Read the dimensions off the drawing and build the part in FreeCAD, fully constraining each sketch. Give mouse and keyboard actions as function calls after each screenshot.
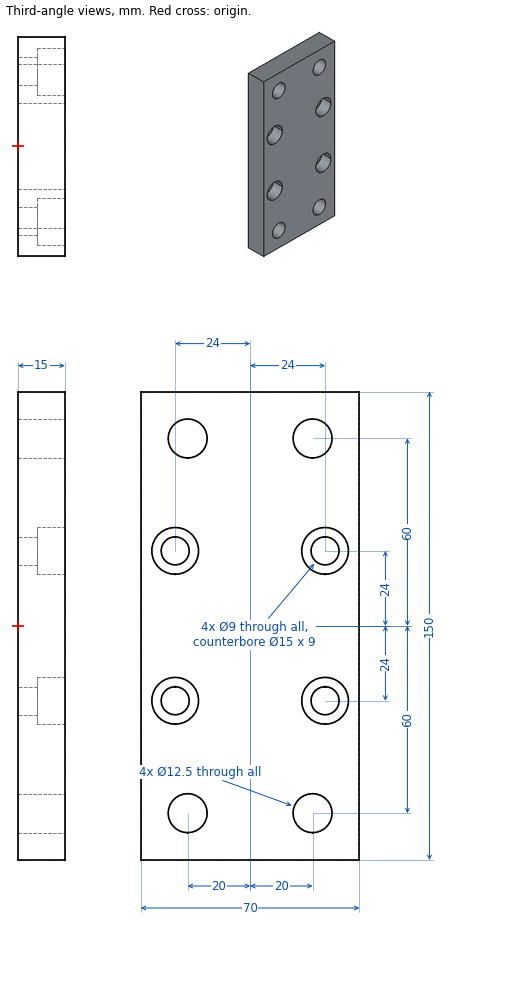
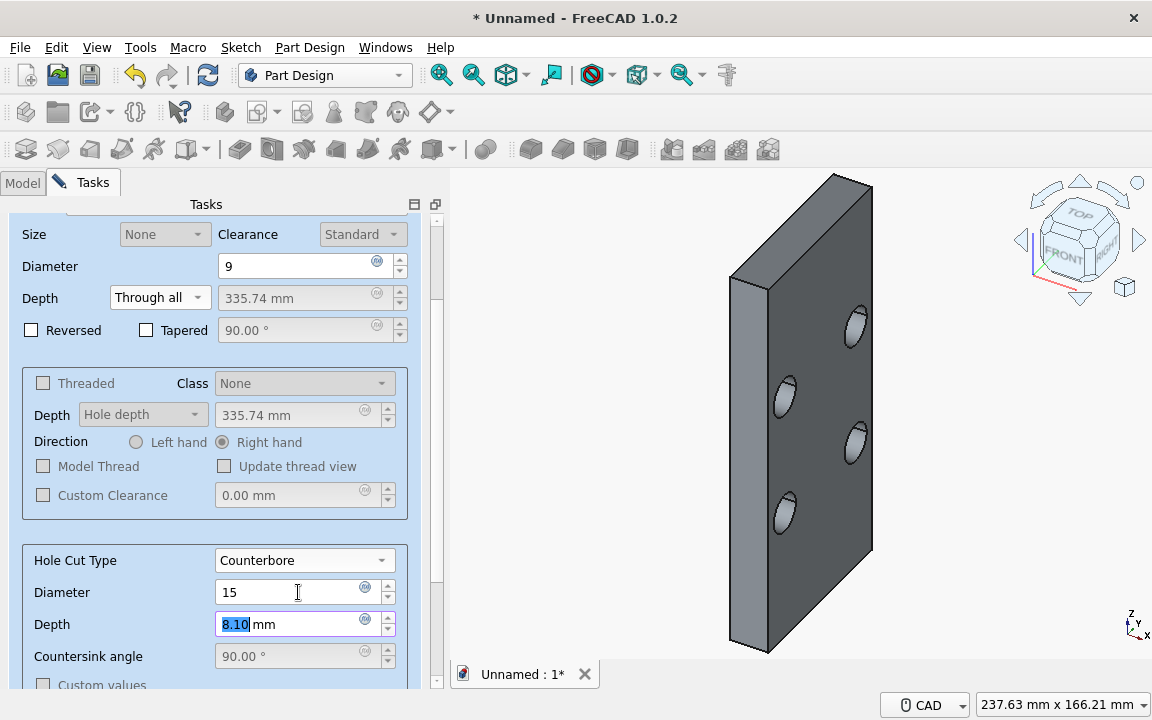
text(9)
key(Tab)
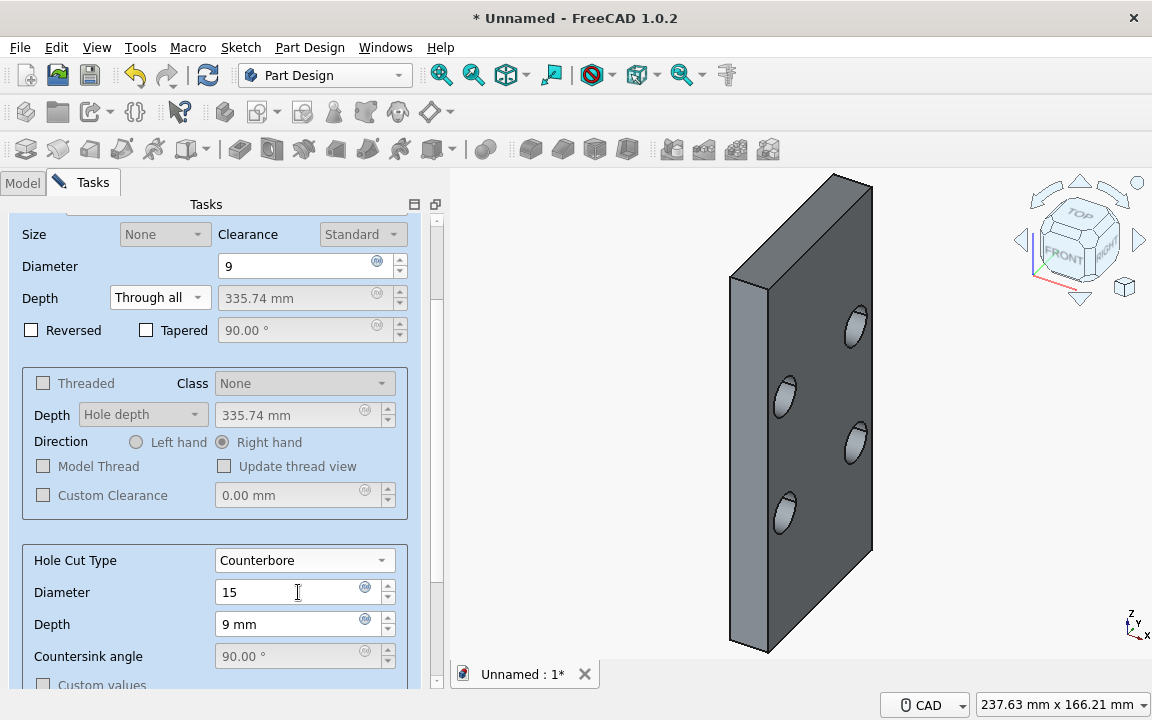
scroll(437, 451, up, 3)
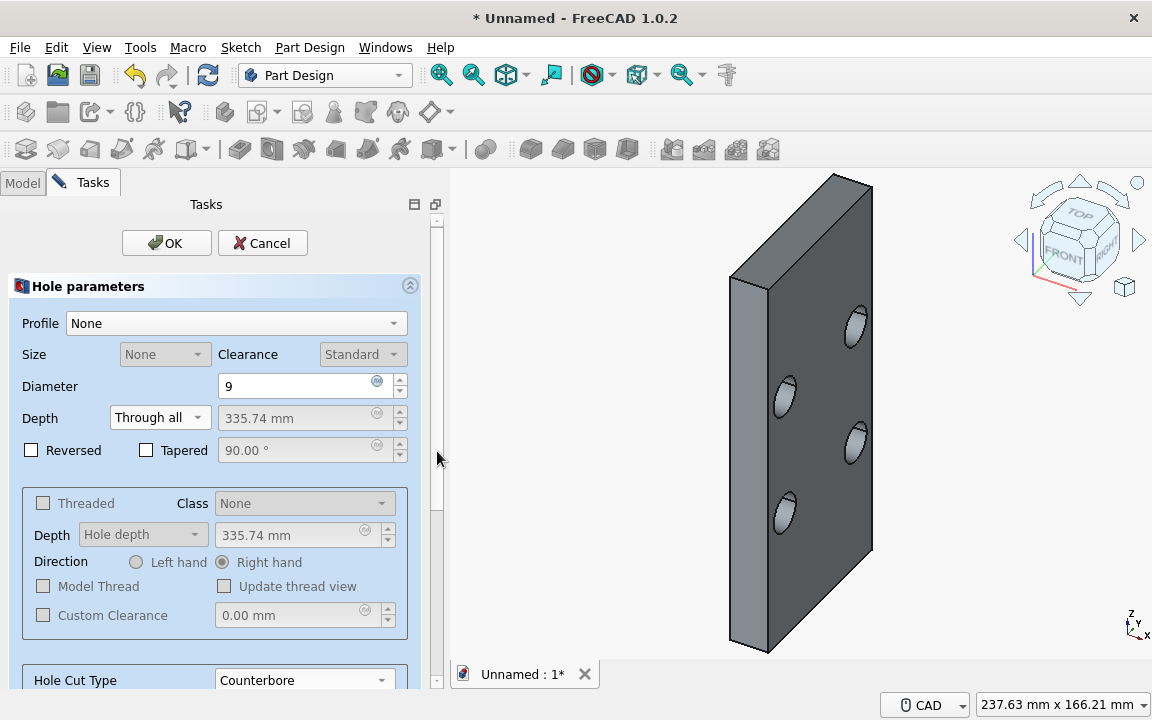
click(167, 243)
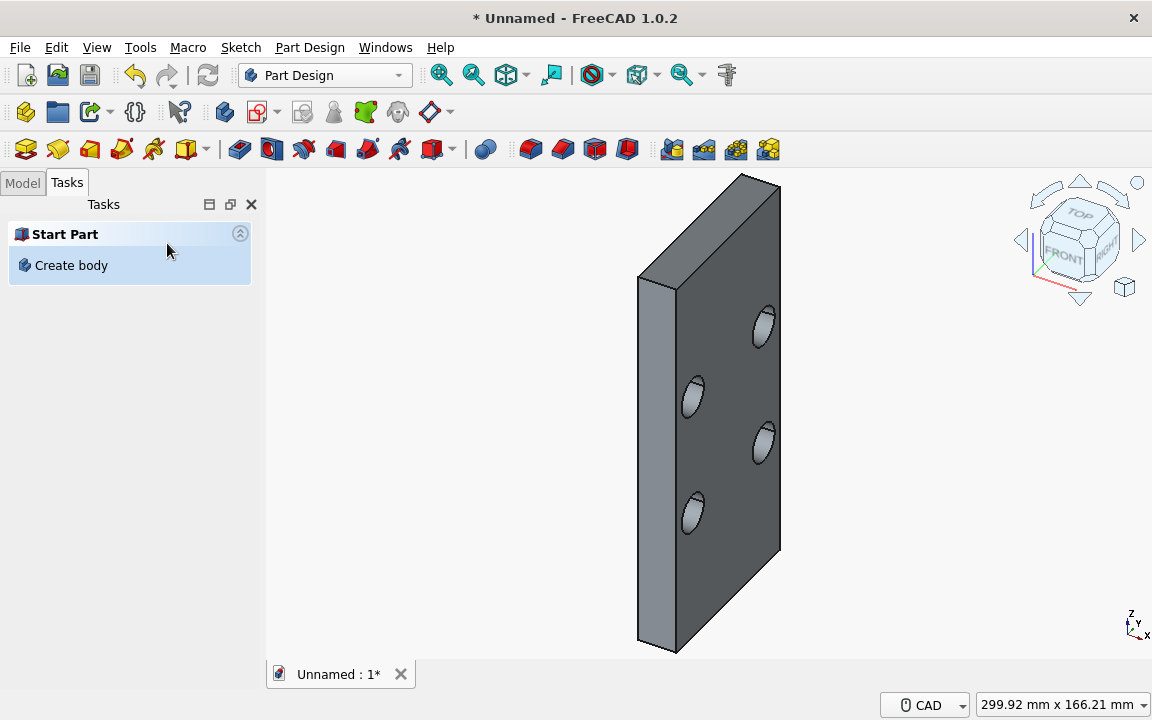
click(258, 112)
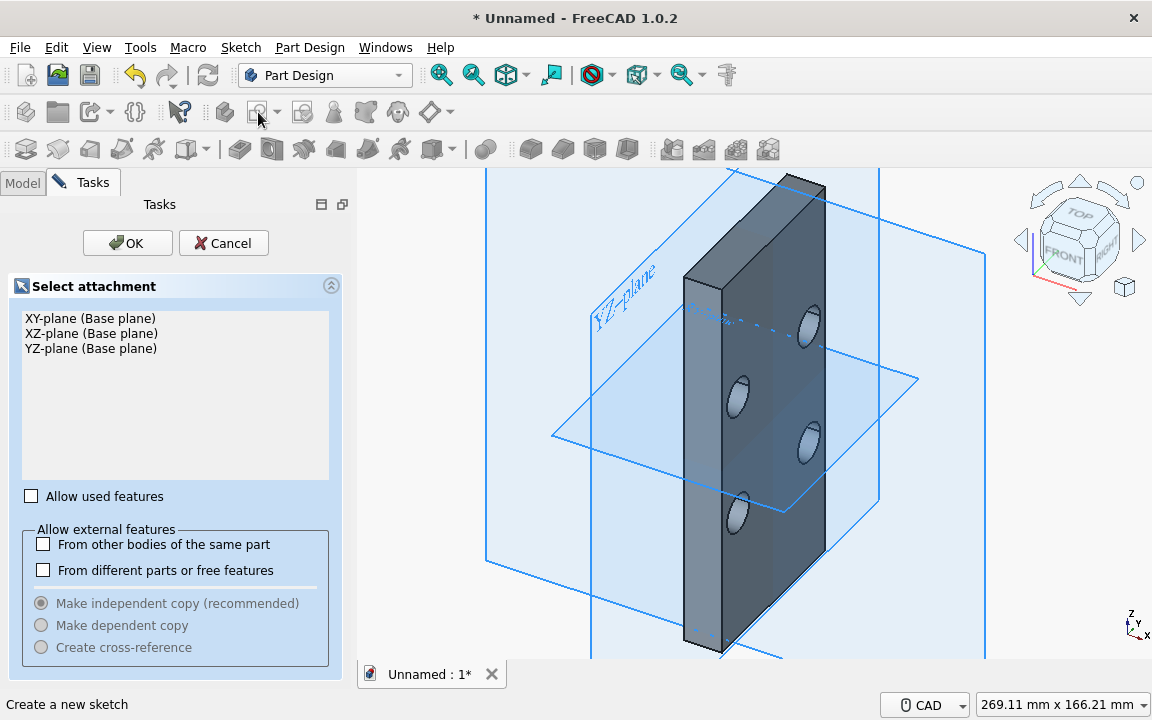
click(82, 348)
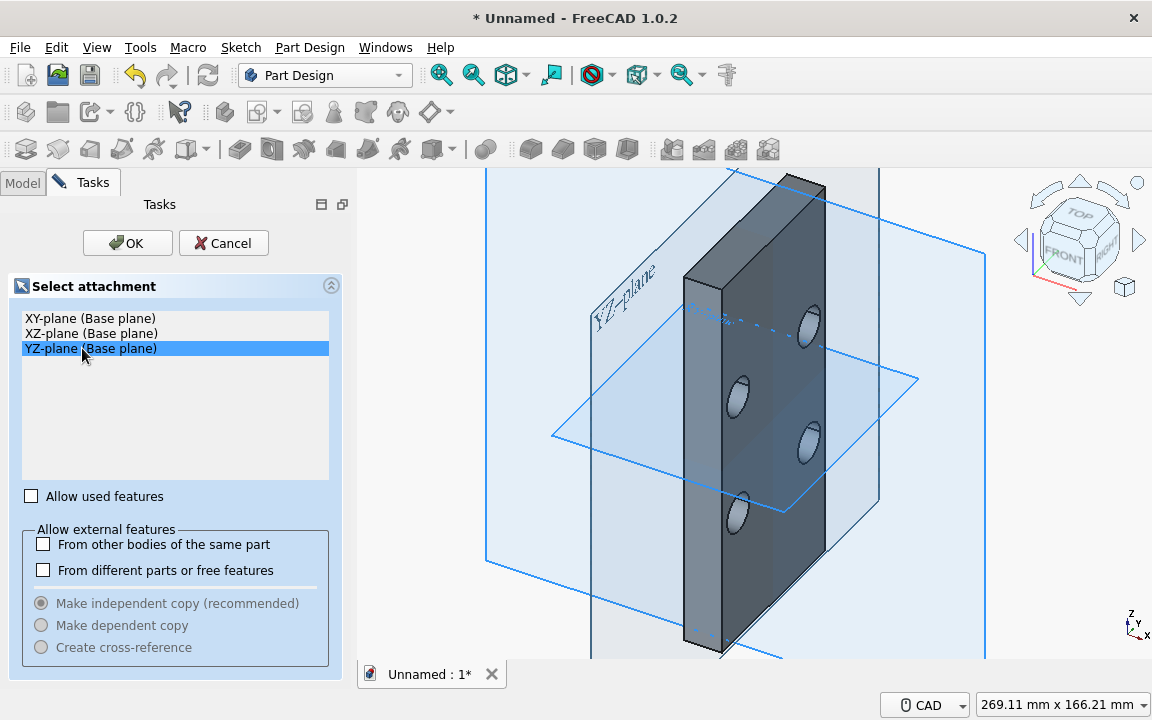
click(128, 243)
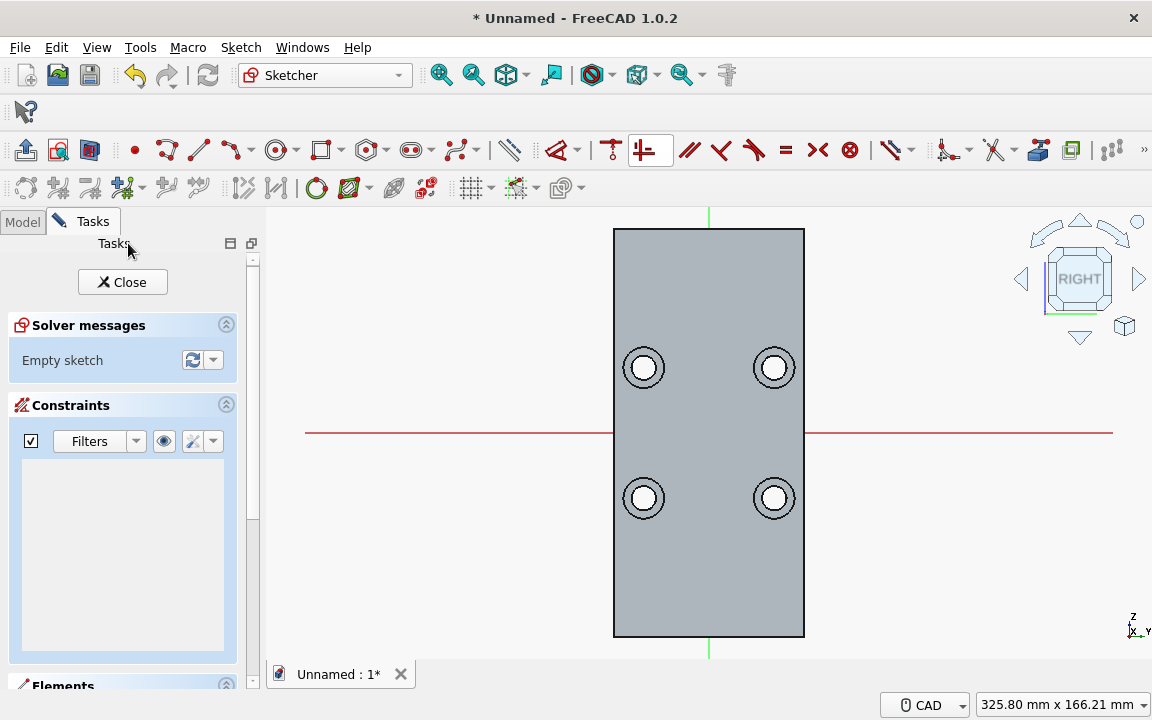
click(90, 150)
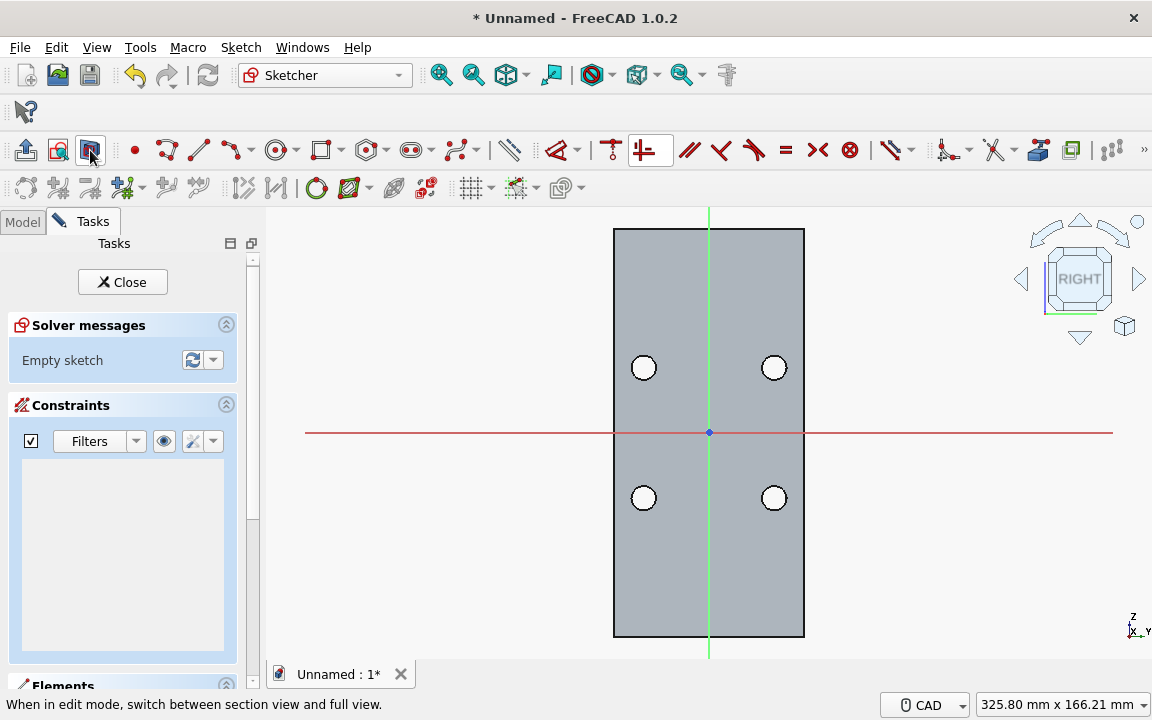
scroll(331, 433, down, 1)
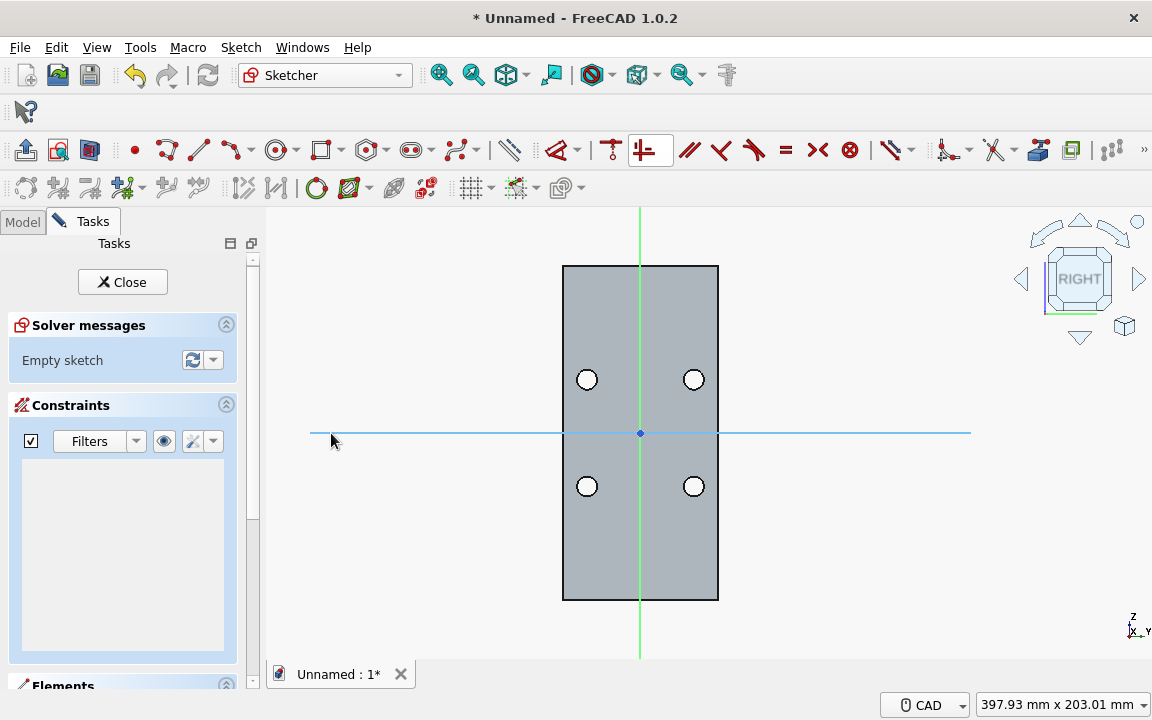
click(276, 150)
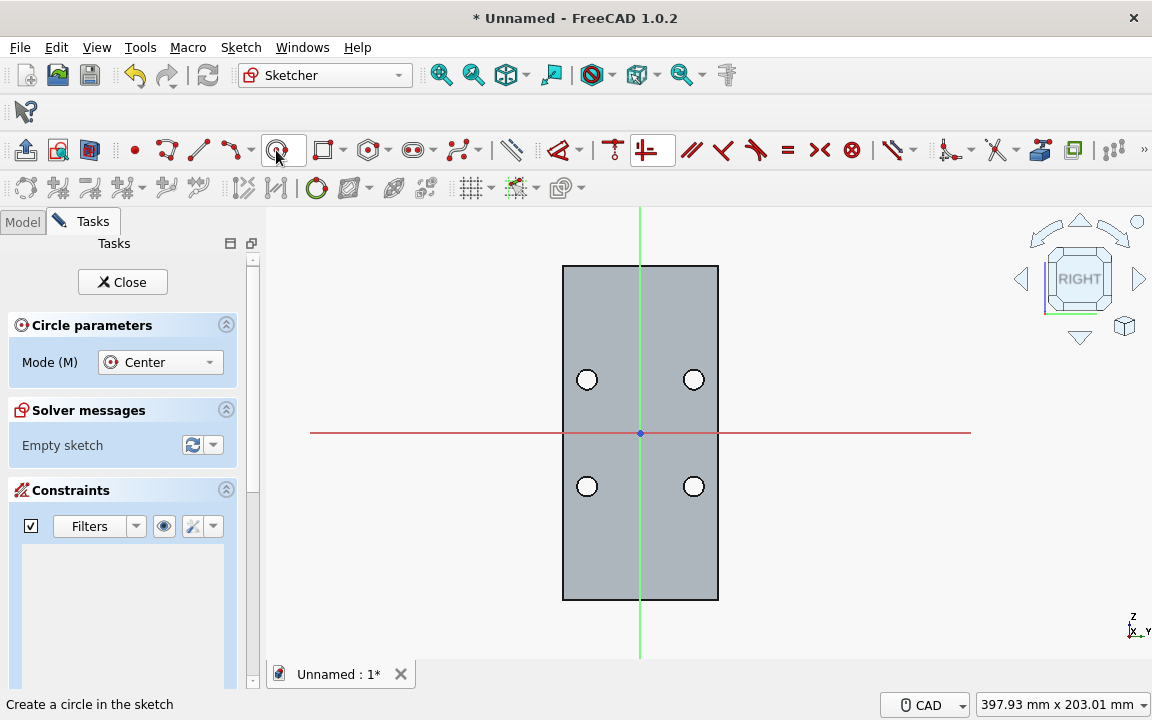
scroll(685, 567, up, 3)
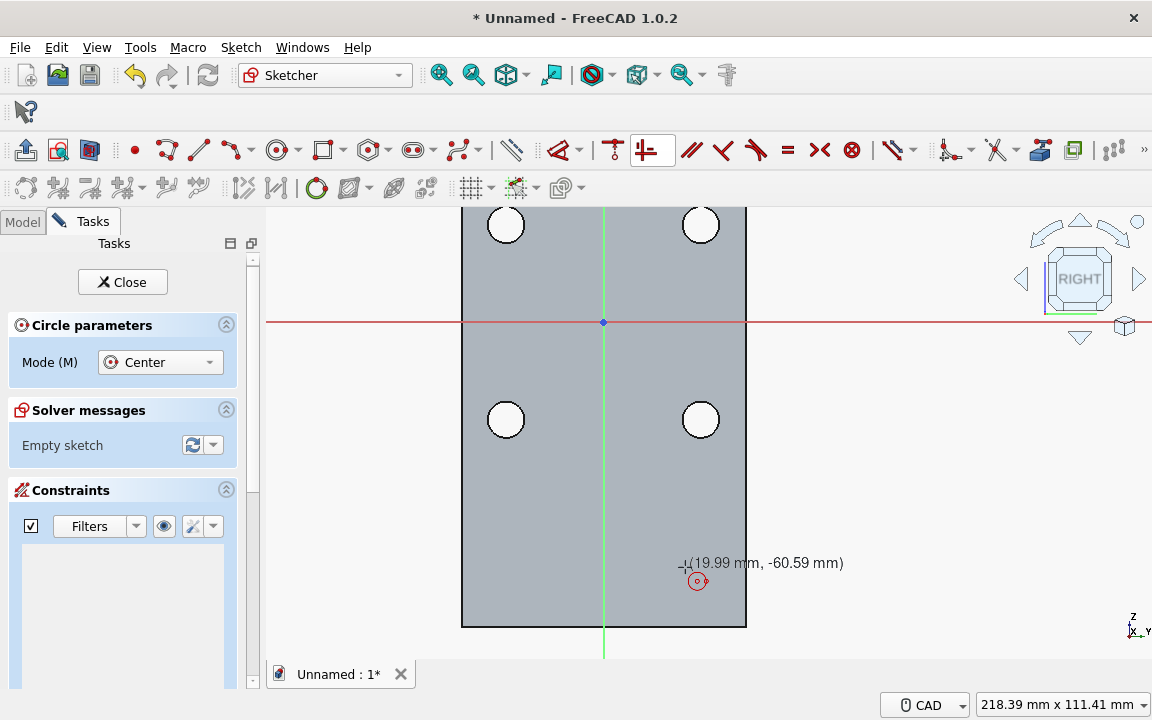
click(685, 566)
click(703, 548)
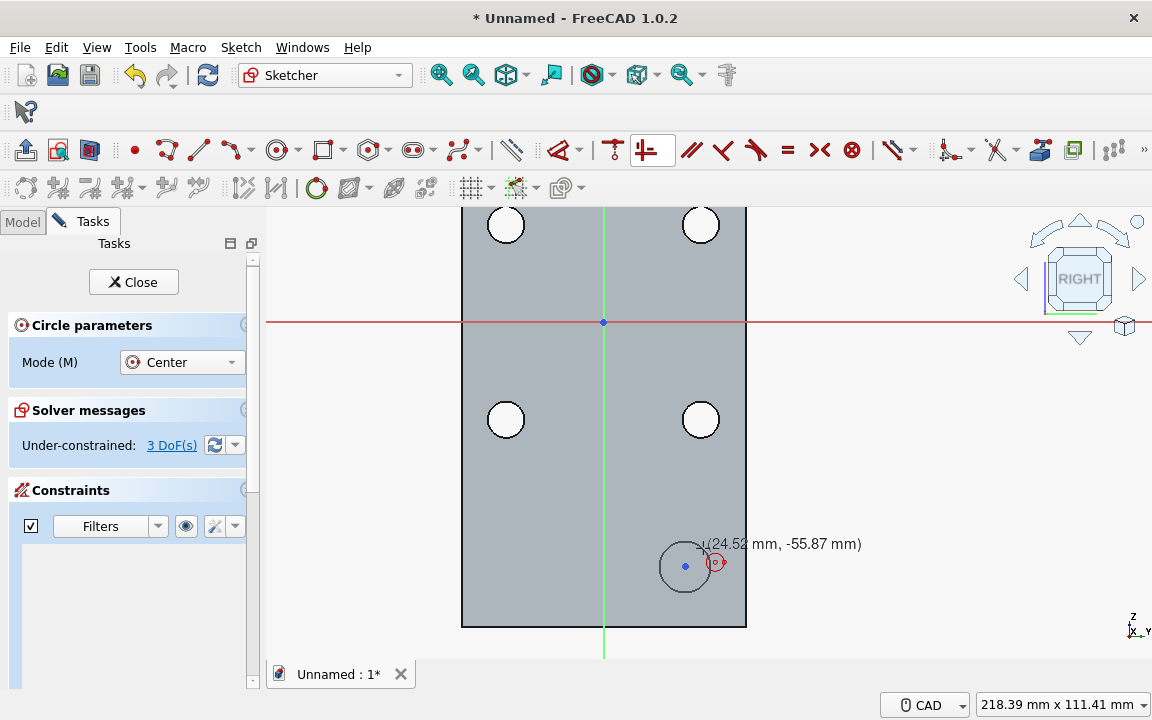
click(522, 566)
click(540, 548)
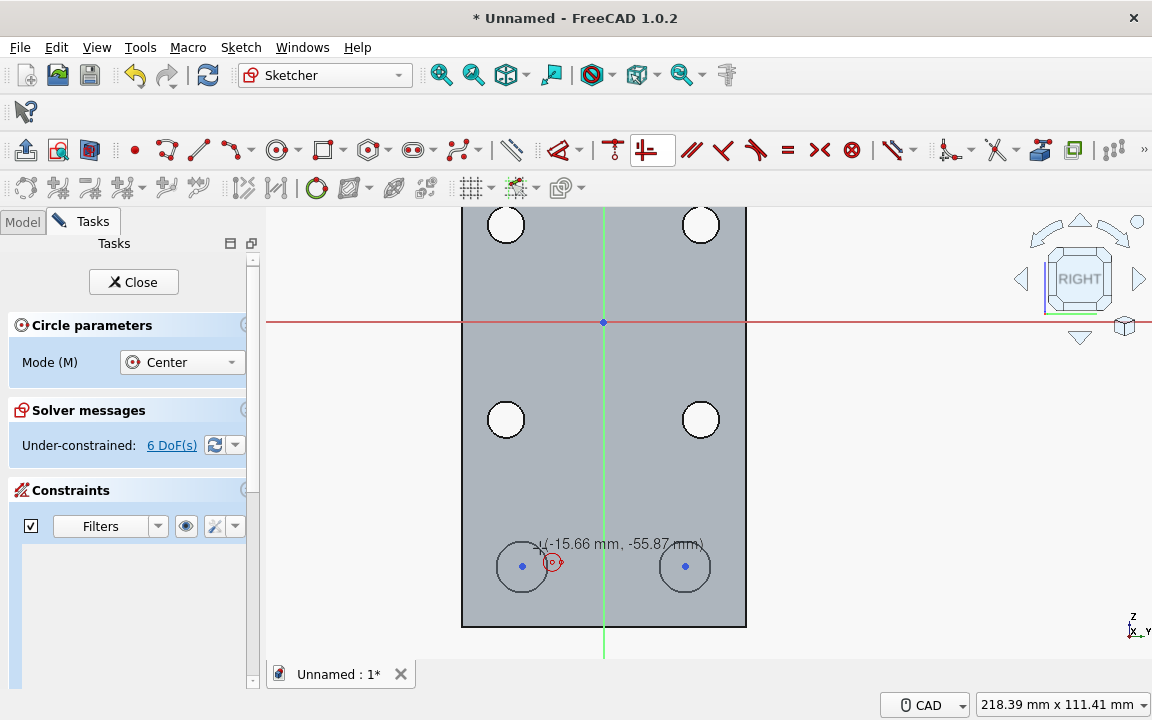
scroll(685, 568, down, 3)